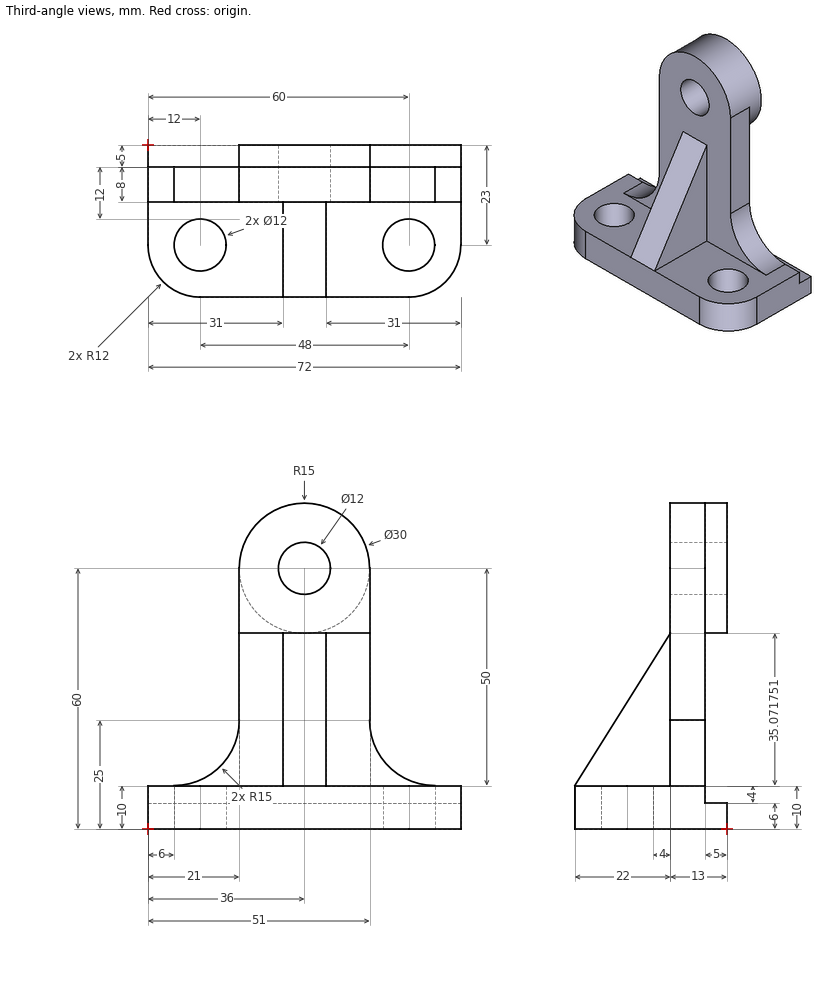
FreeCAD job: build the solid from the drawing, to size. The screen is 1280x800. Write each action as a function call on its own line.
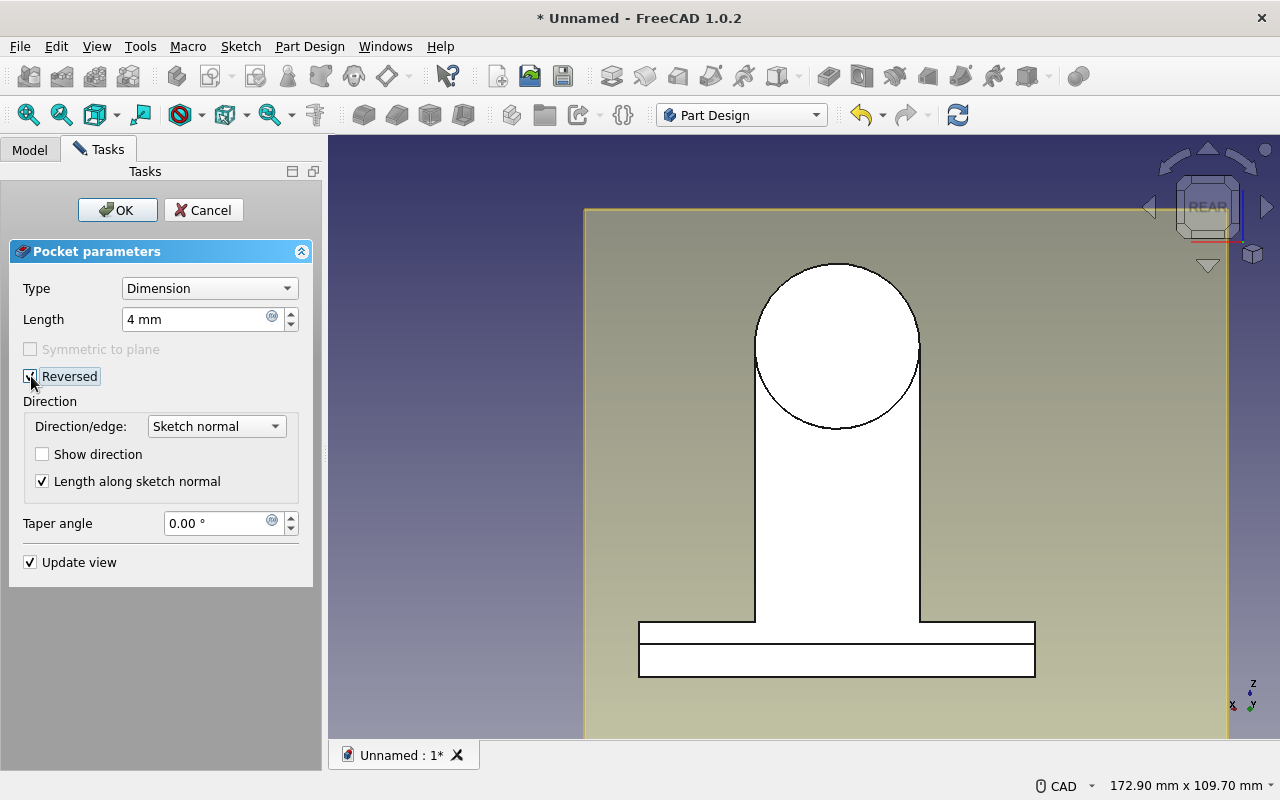
click(118, 210)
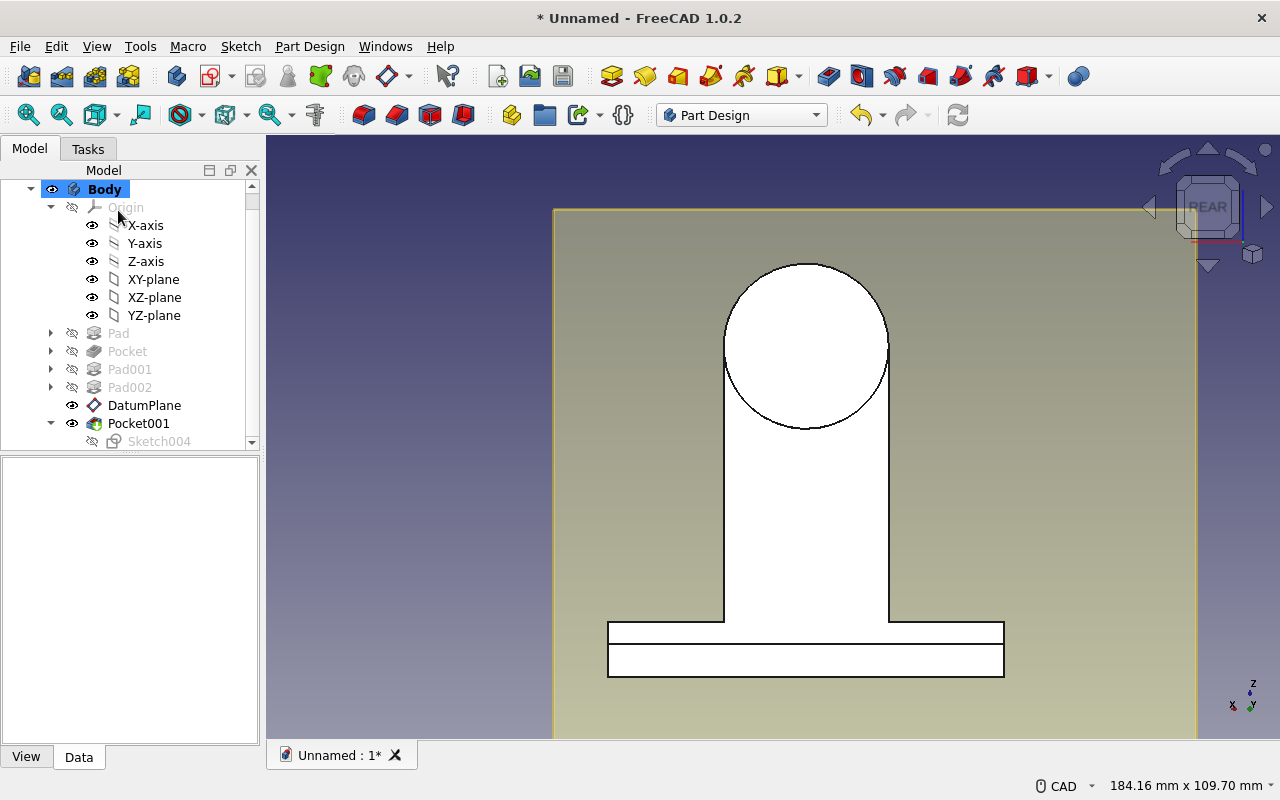
click(117, 405)
key(space)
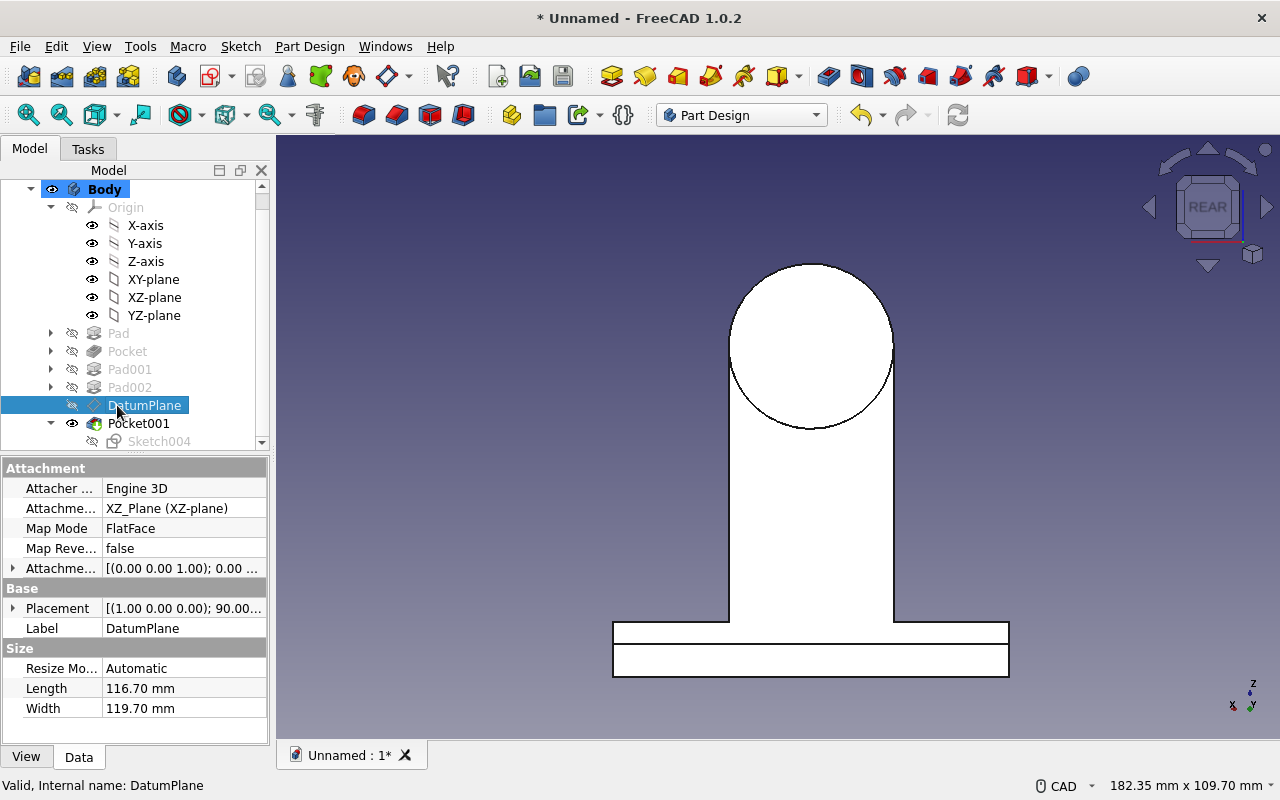
key(0)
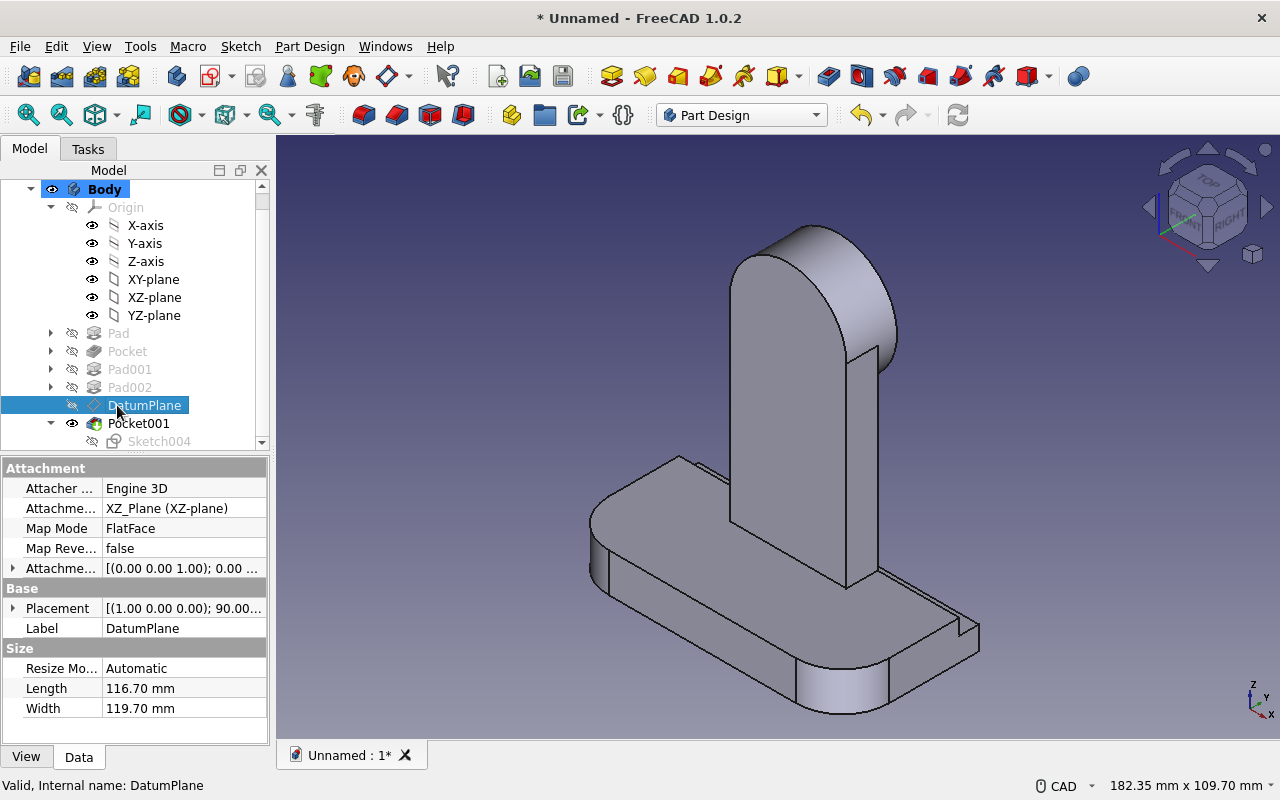
click(788, 366)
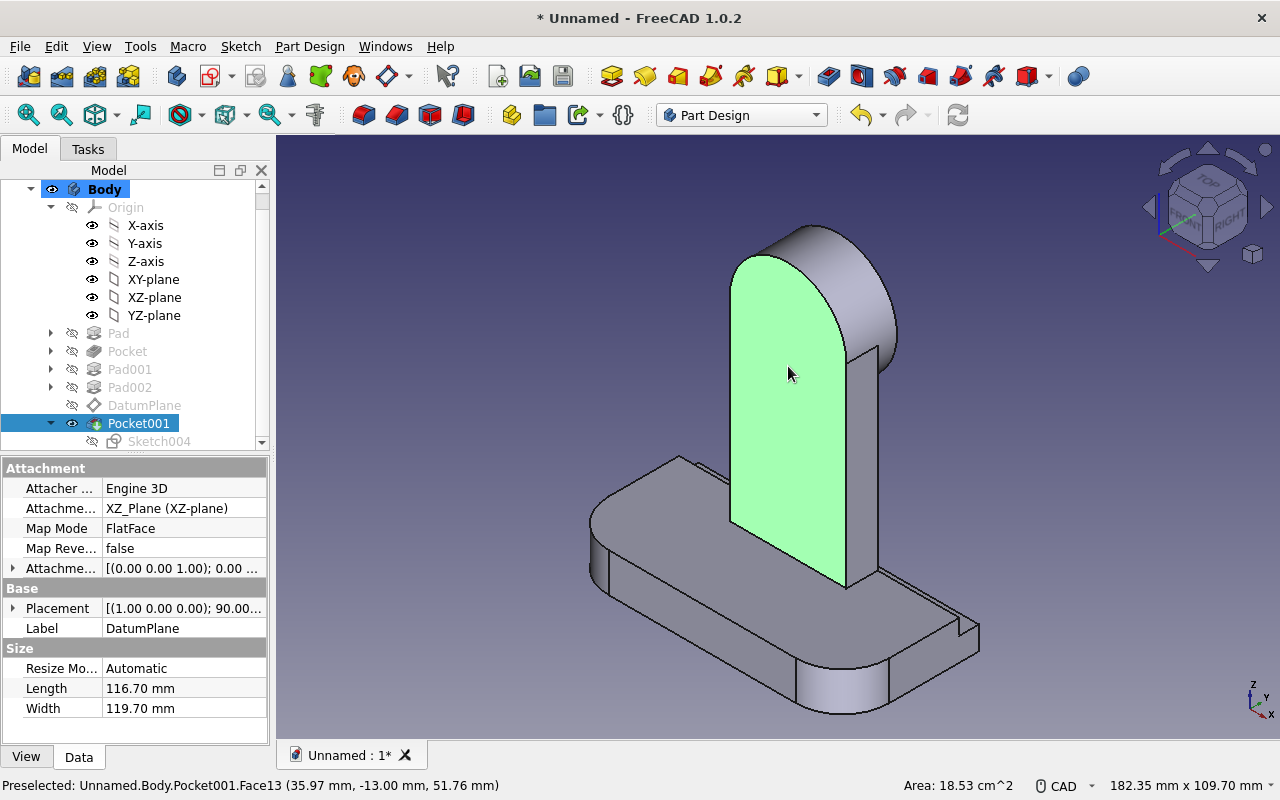
click(210, 76)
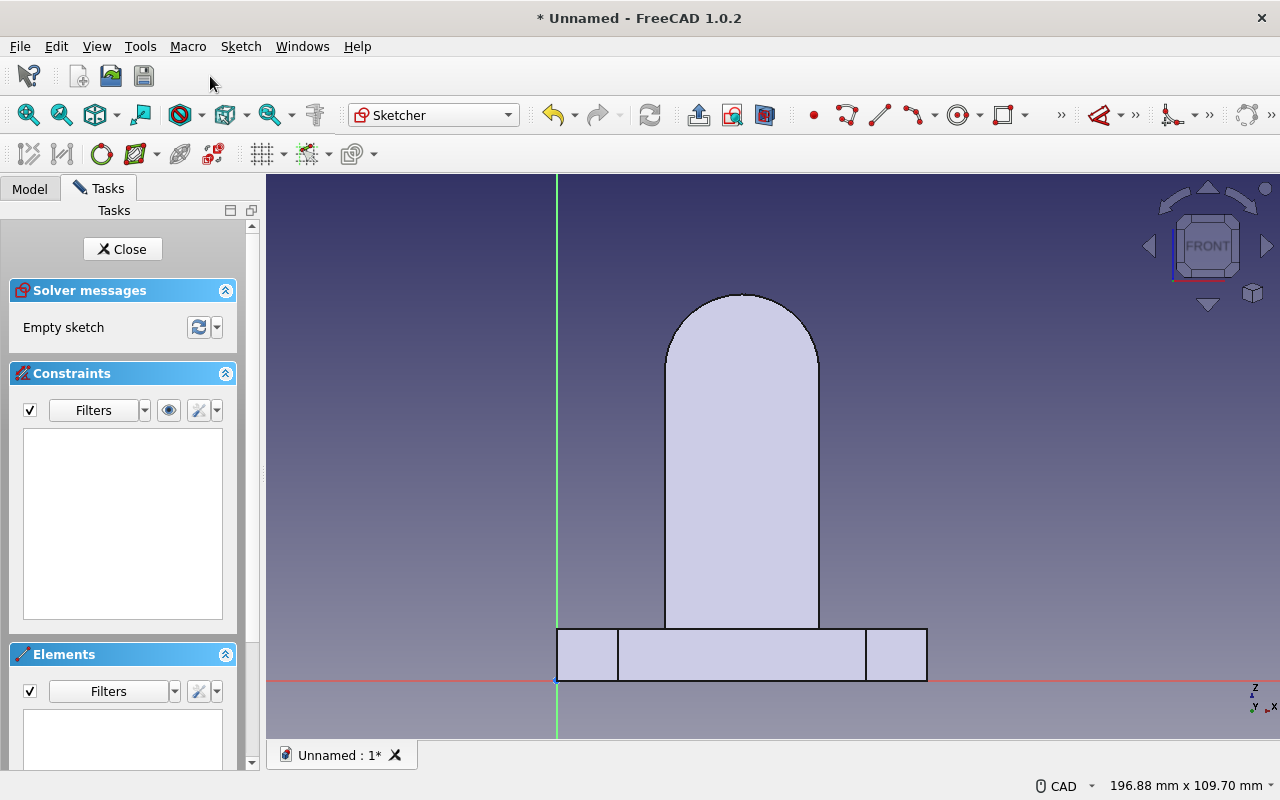
key(q)
key(s)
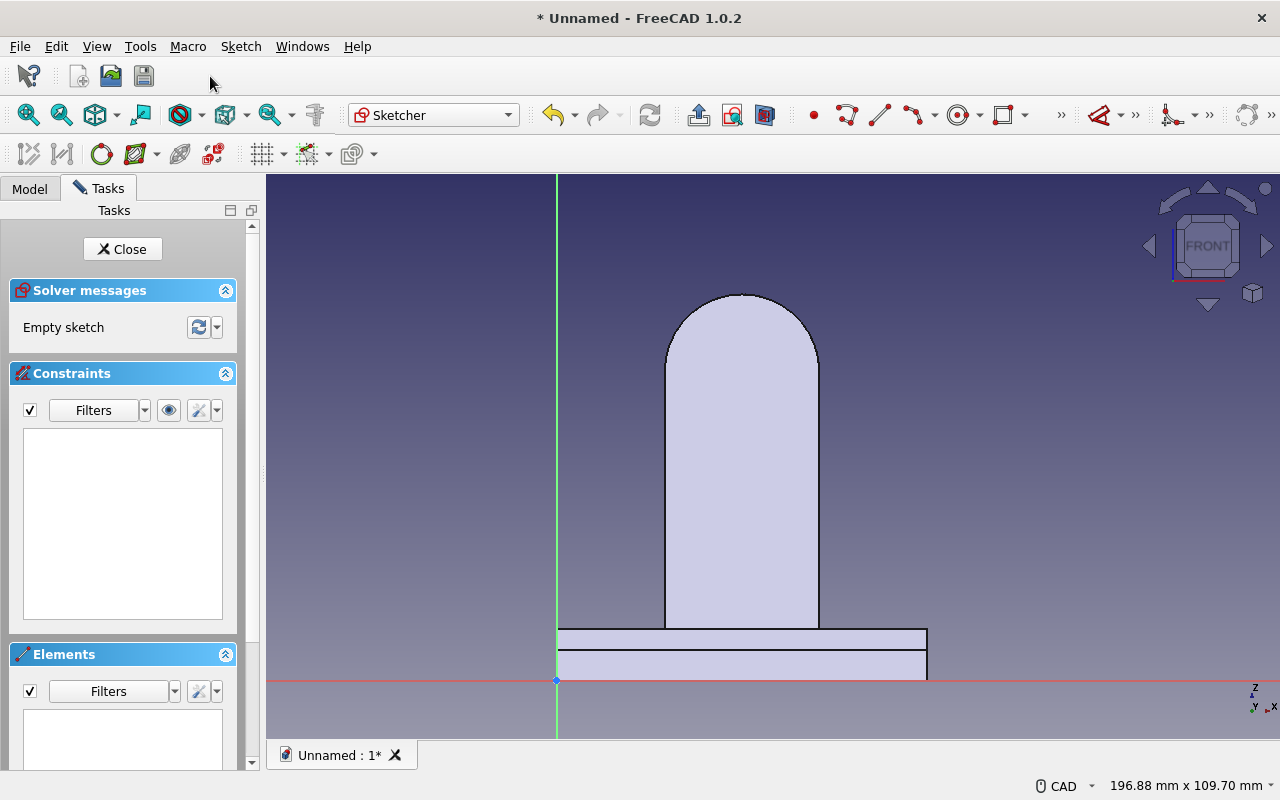
scroll(749, 355, up, 9)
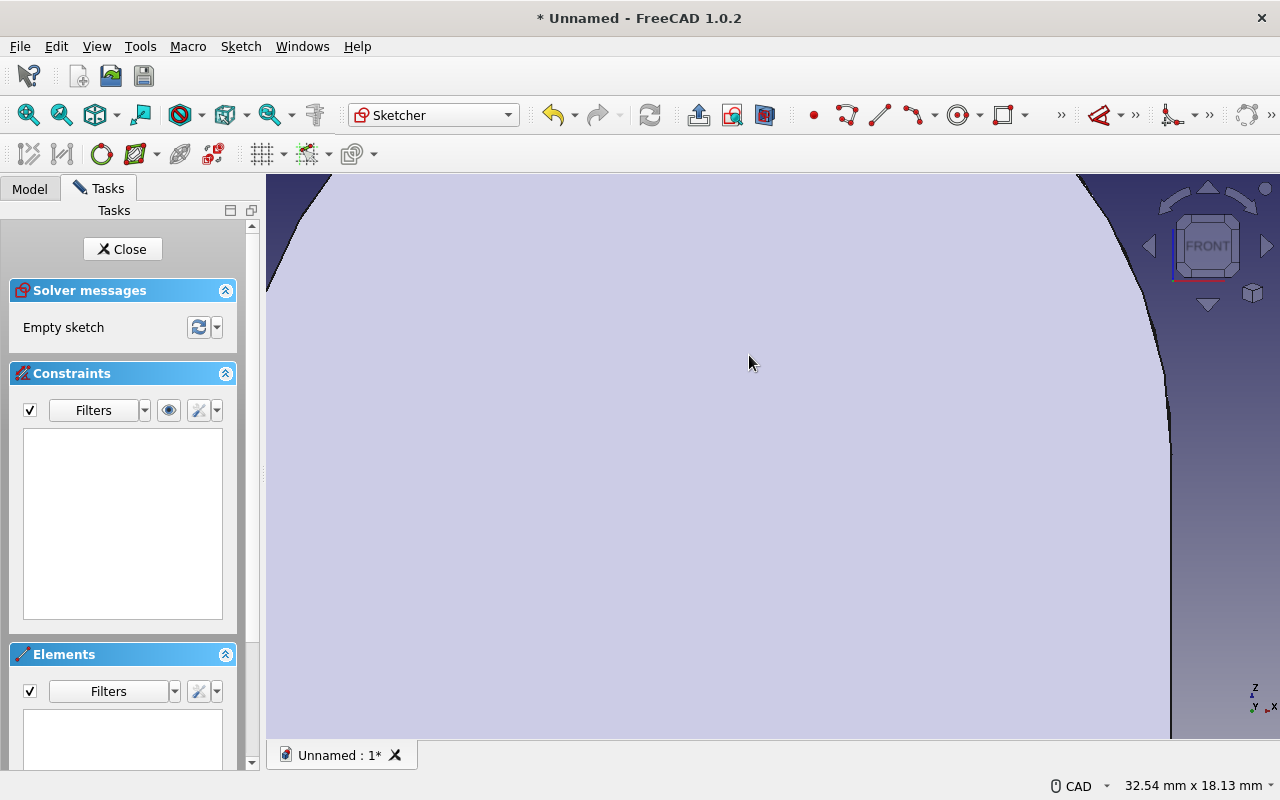
click(958, 116)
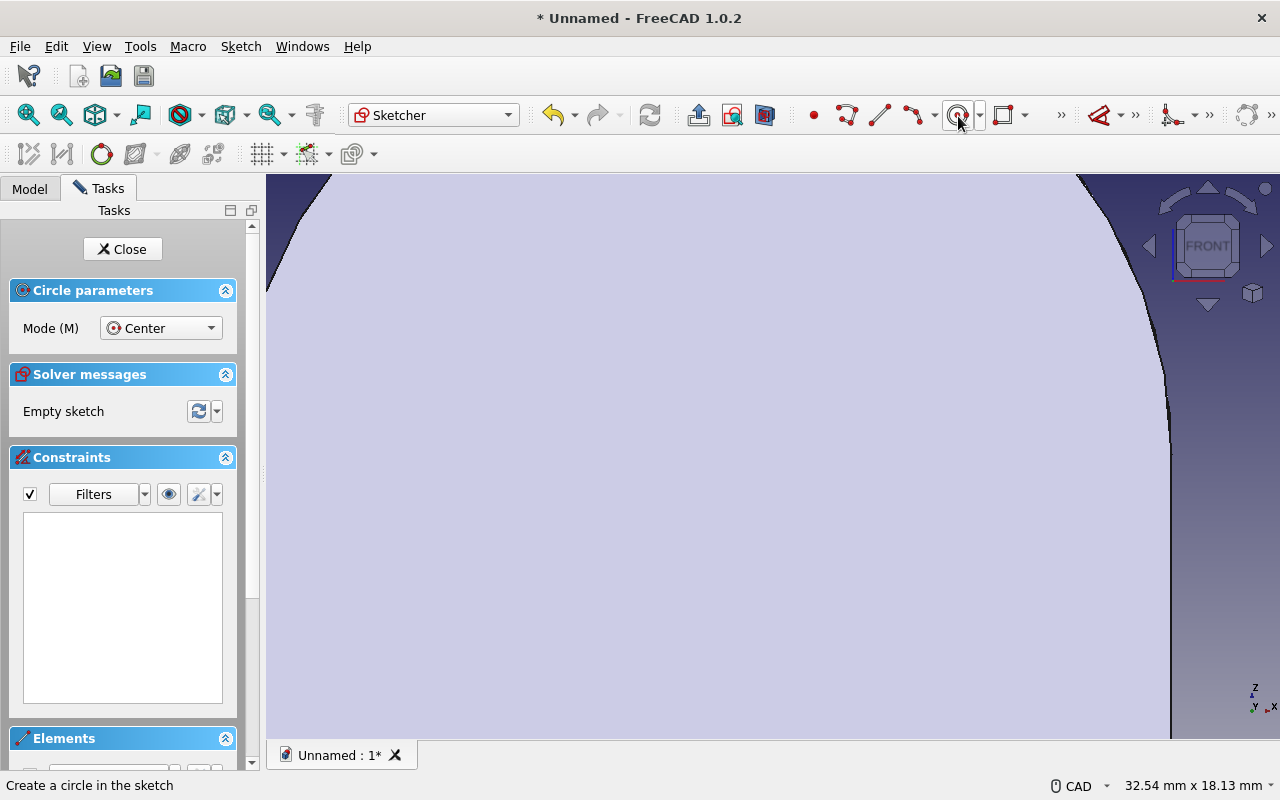
click(704, 454)
click(836, 322)
key(Escape)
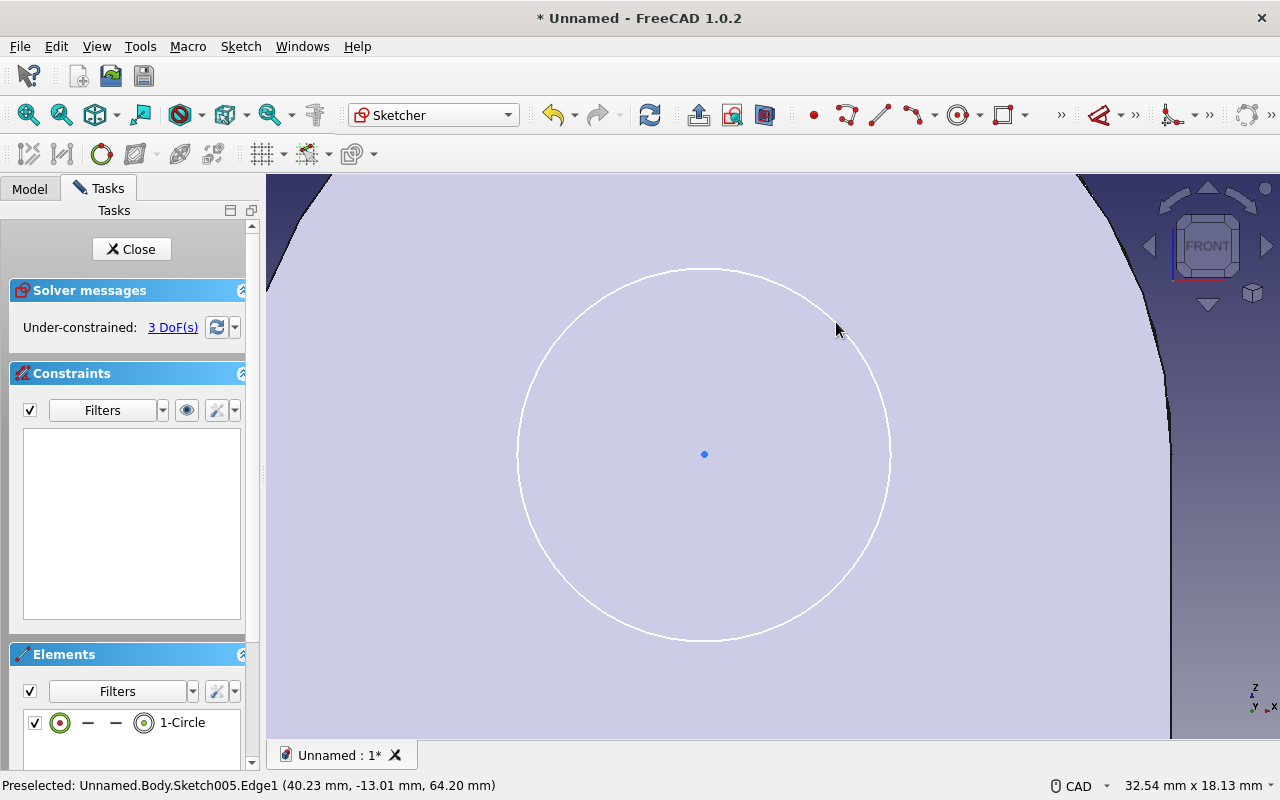
click(1098, 116)